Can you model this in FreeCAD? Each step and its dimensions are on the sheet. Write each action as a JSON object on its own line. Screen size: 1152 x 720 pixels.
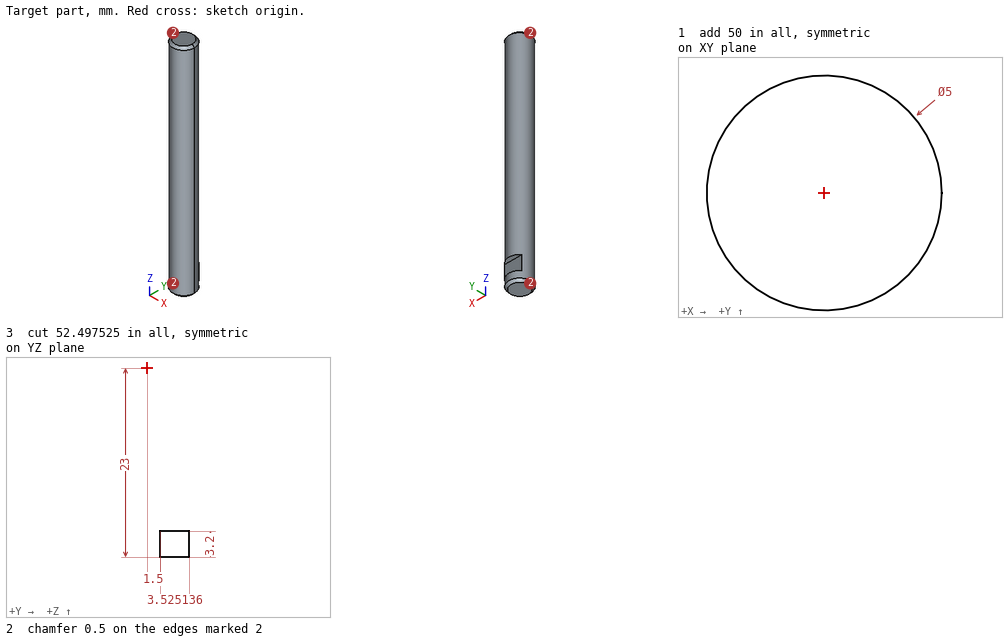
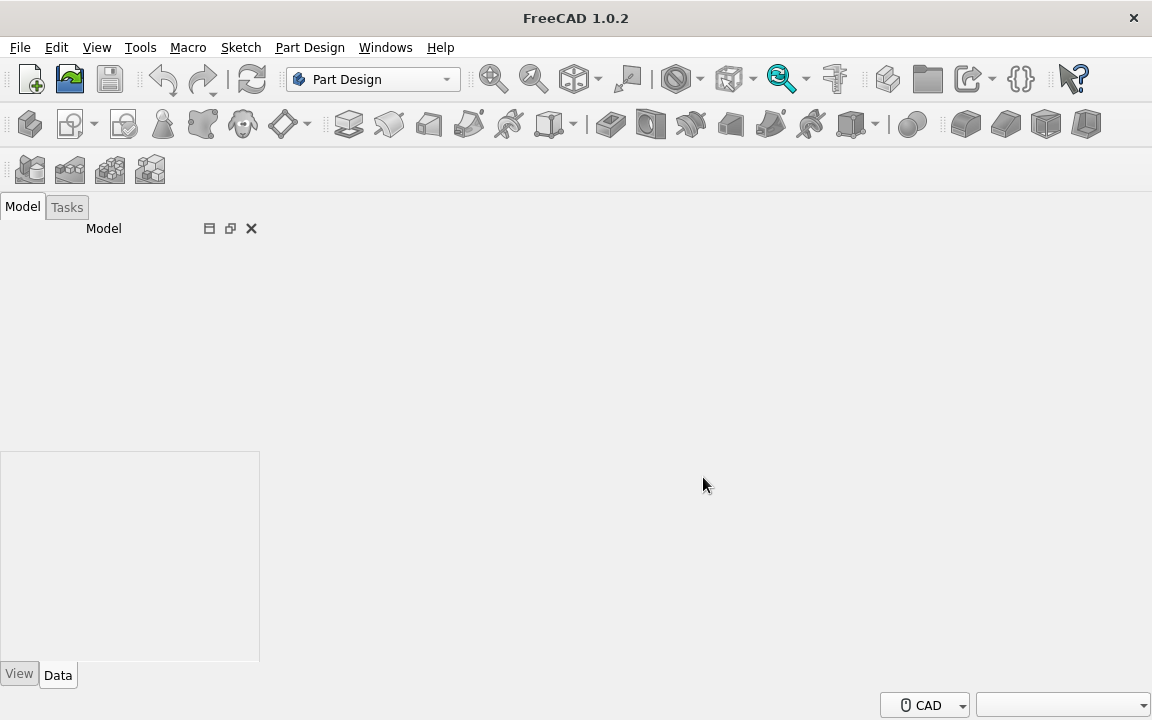
{"action": "left_click", "coordinate": [30, 80]}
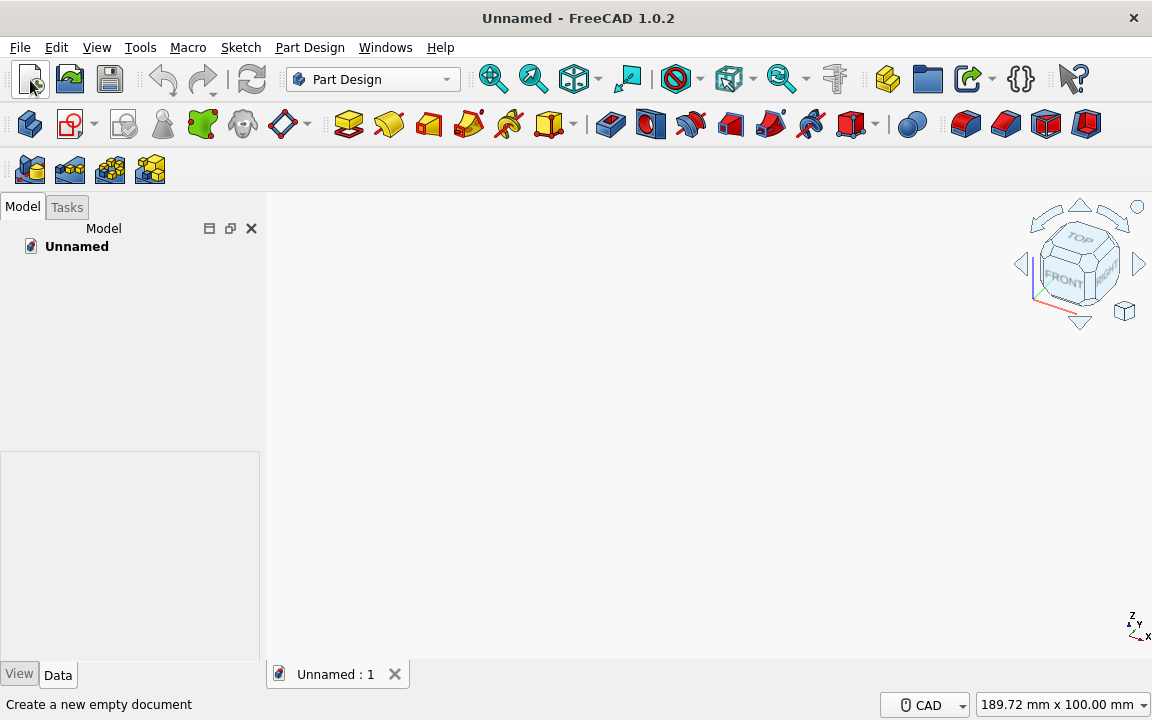
{"action": "left_click", "coordinate": [70, 124]}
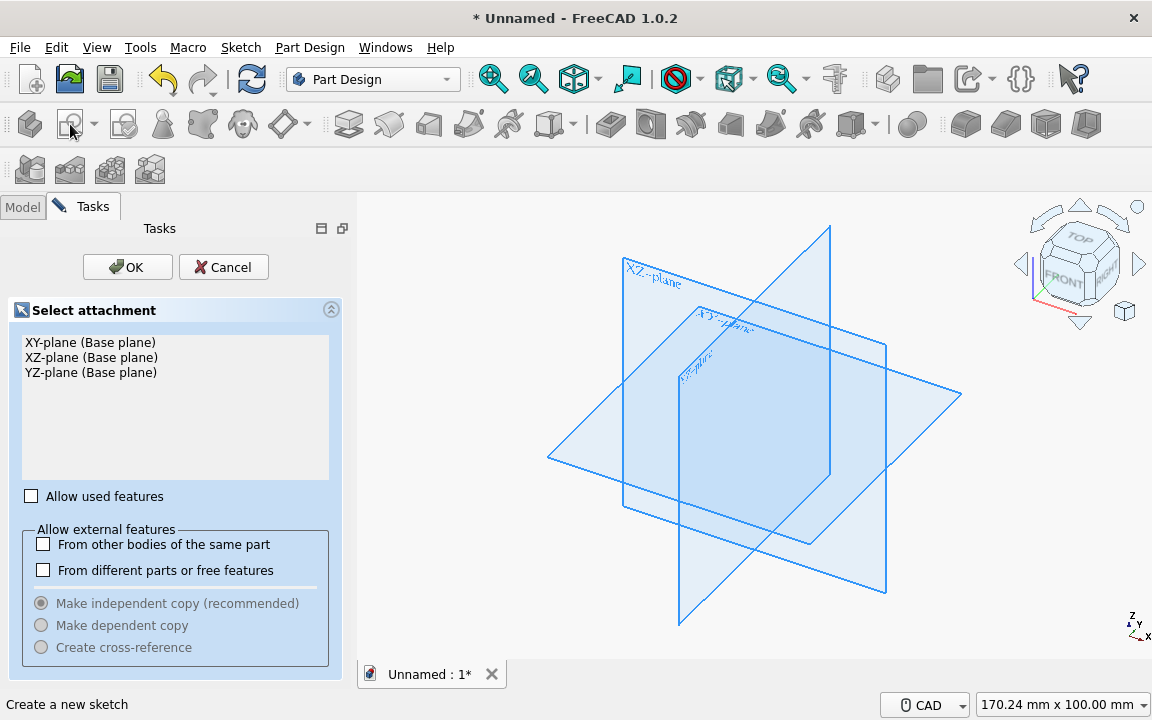
{"action": "left_click", "coordinate": [82, 342]}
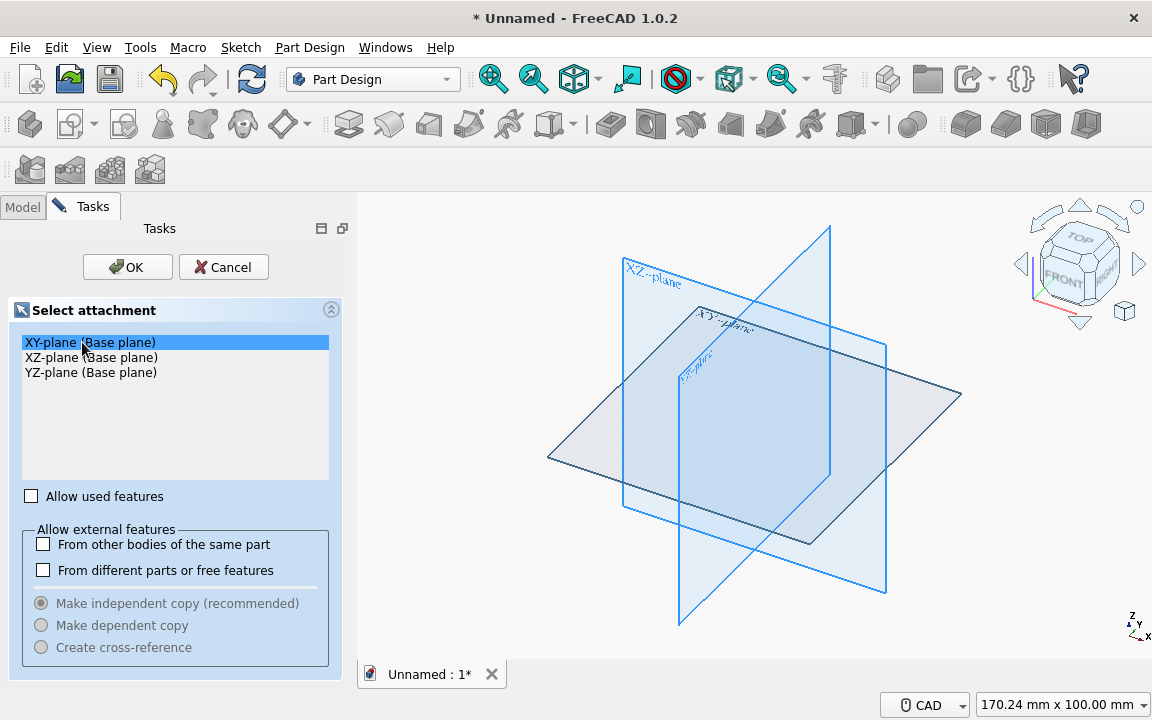
{"action": "left_click", "coordinate": [128, 267]}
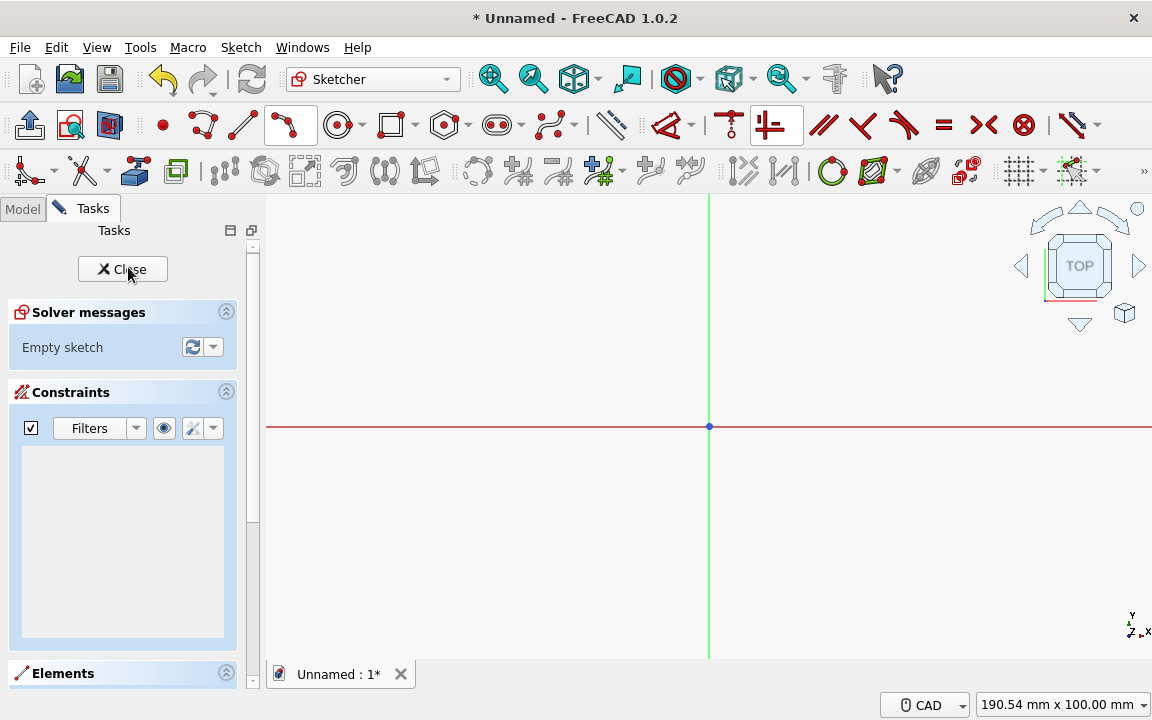
{"action": "scroll", "coordinate": [714, 426], "scroll_direction": "up", "scroll_amount": 13}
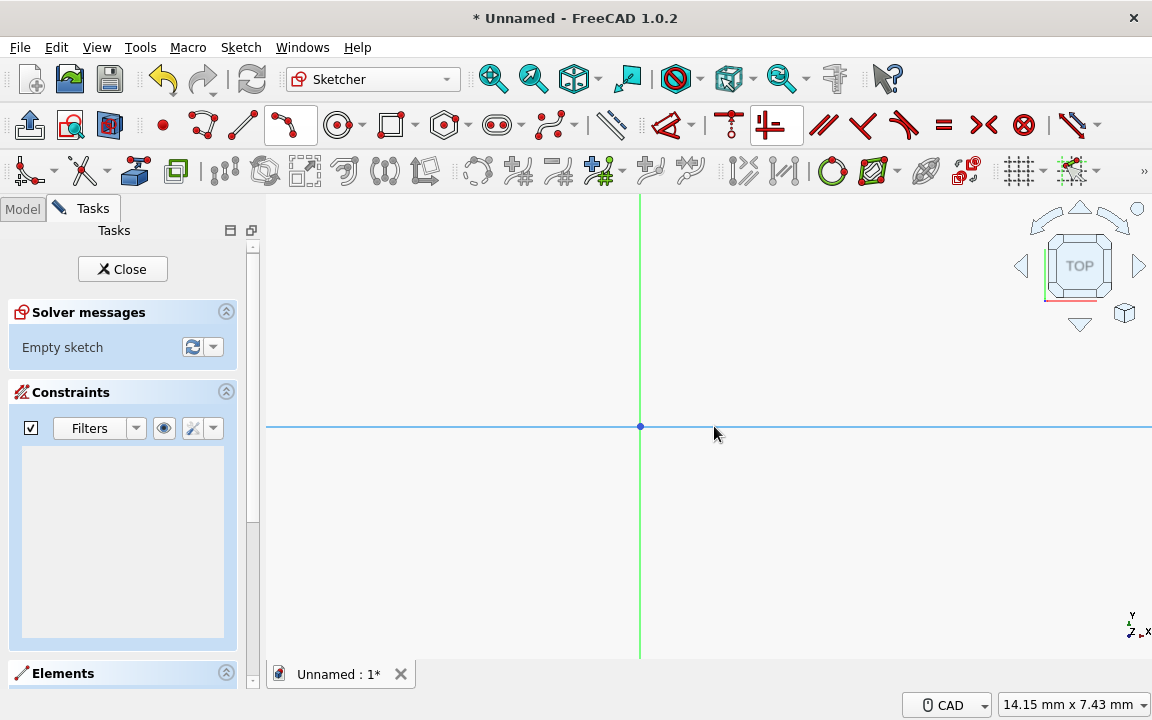
{"action": "key", "text": "g c"}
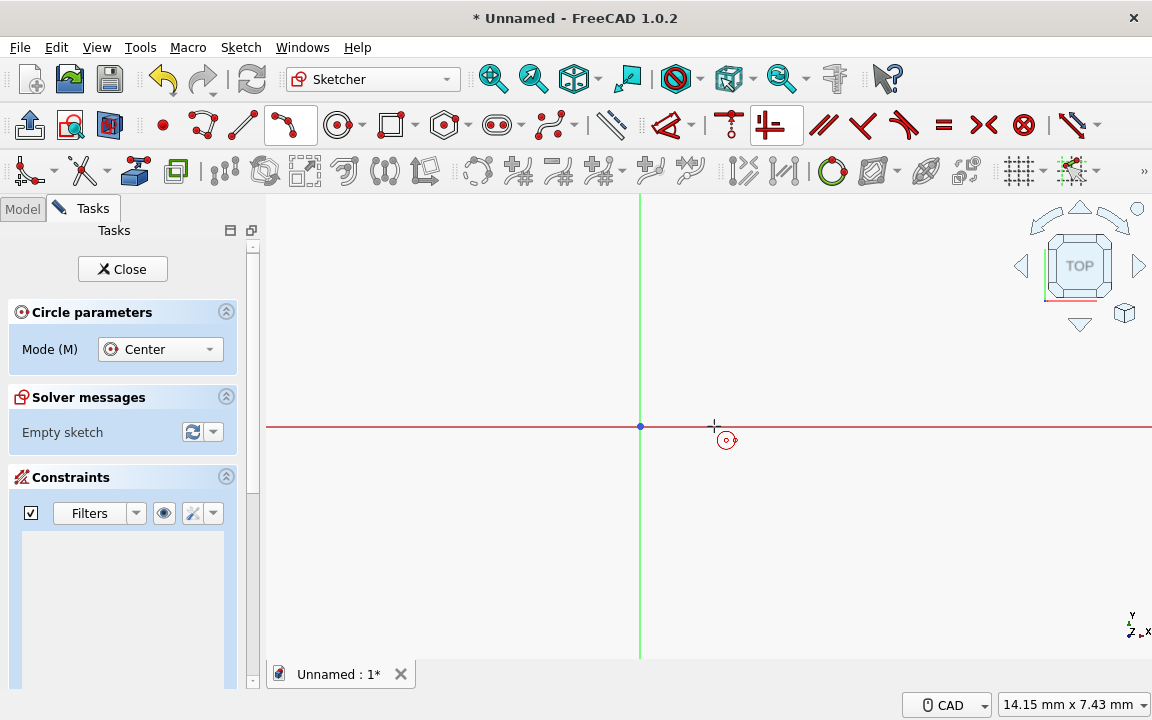
{"action": "left_click", "coordinate": [640, 426]}
{"action": "mouse_move", "coordinate": [751, 316]}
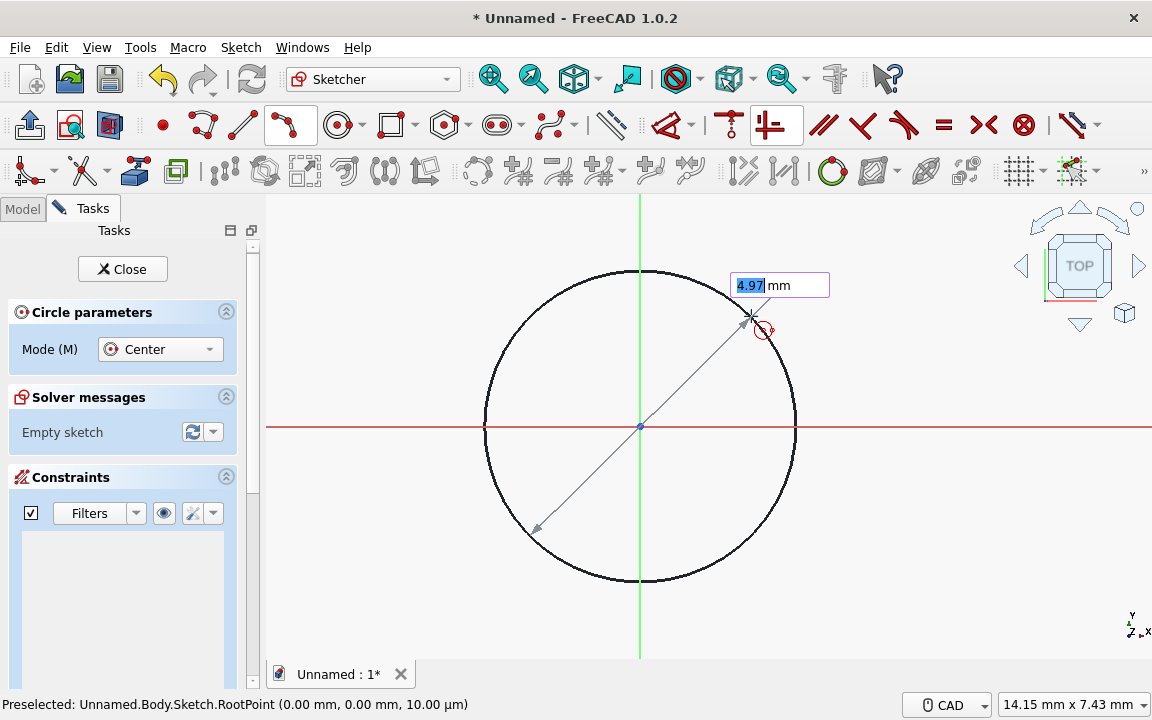
{"action": "type", "text": "5"}
{"action": "key", "text": "Return"}
{"action": "key", "text": "Escape"}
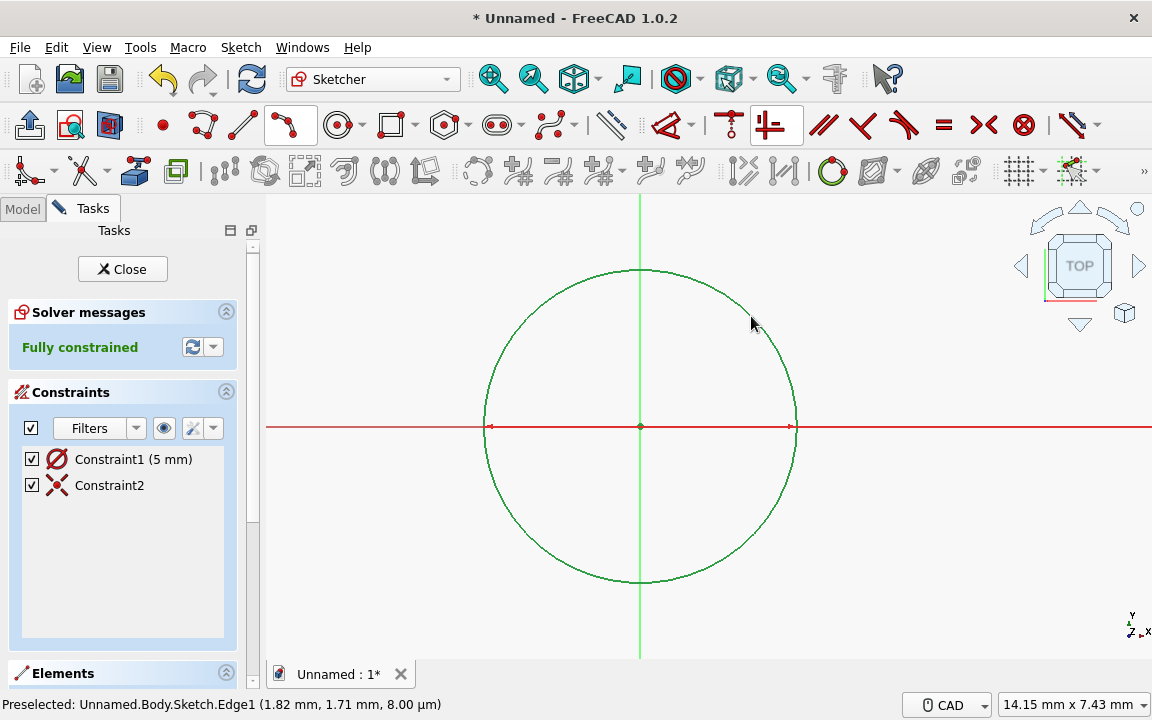
{"action": "left_click", "coordinate": [123, 269]}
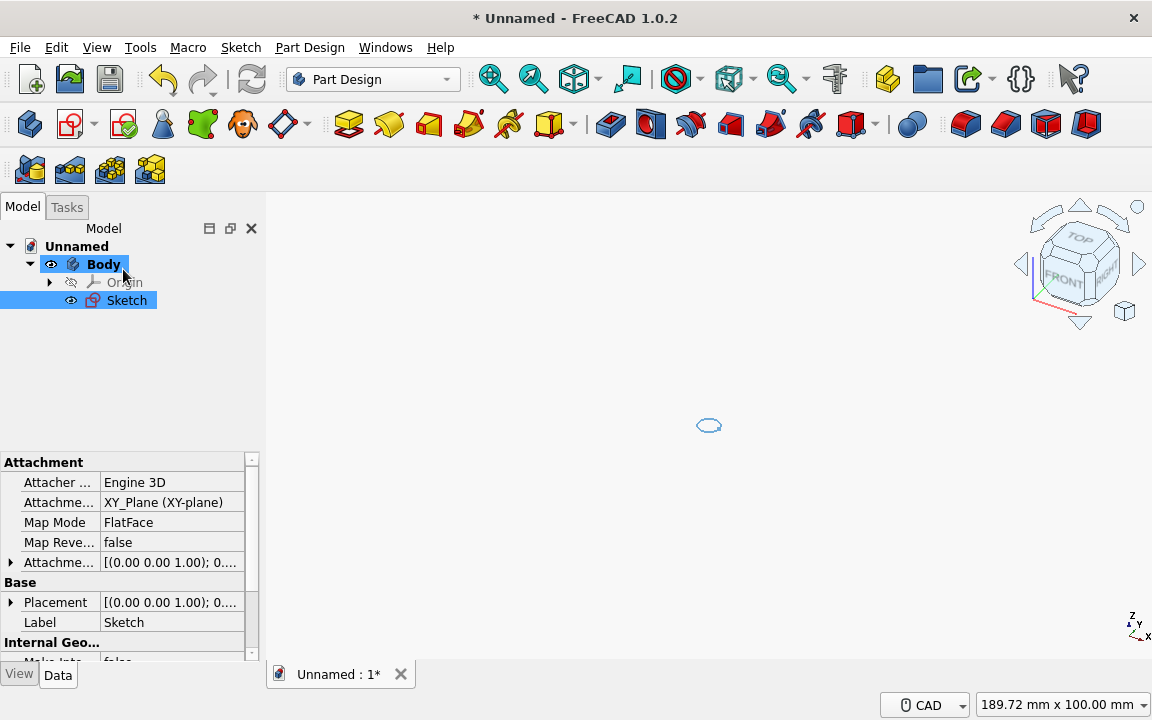
{"action": "left_click", "coordinate": [350, 124]}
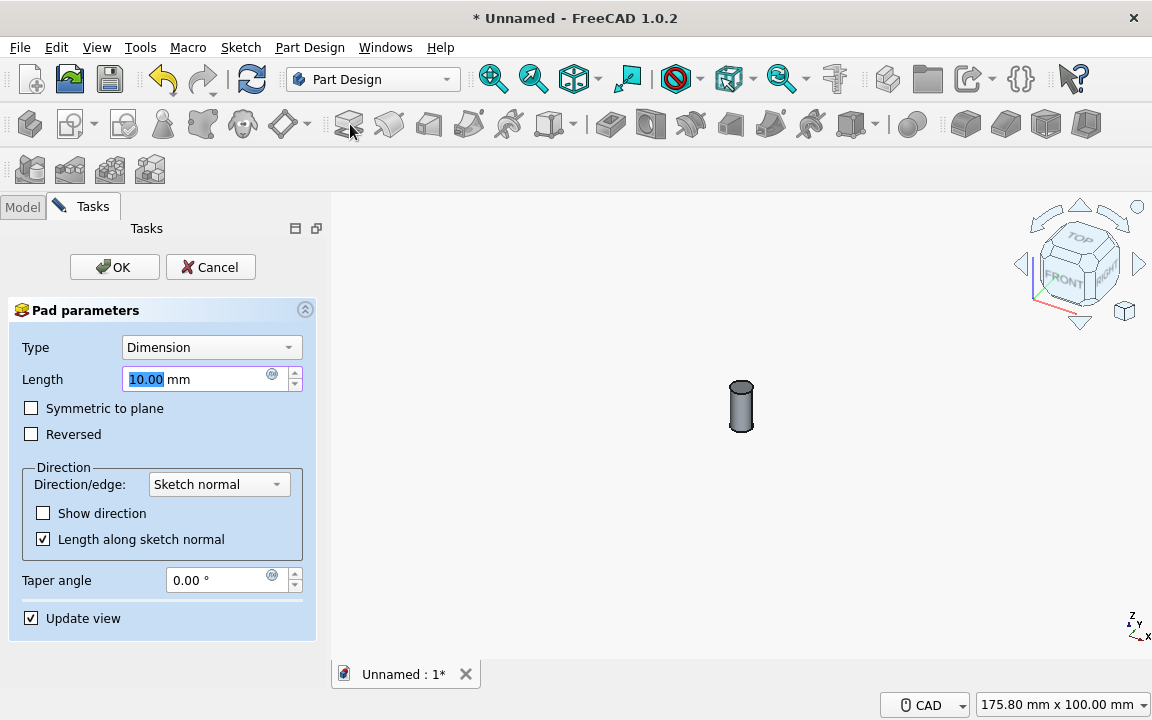
{"action": "type", "text": "50"}
{"action": "key", "text": "Tab"}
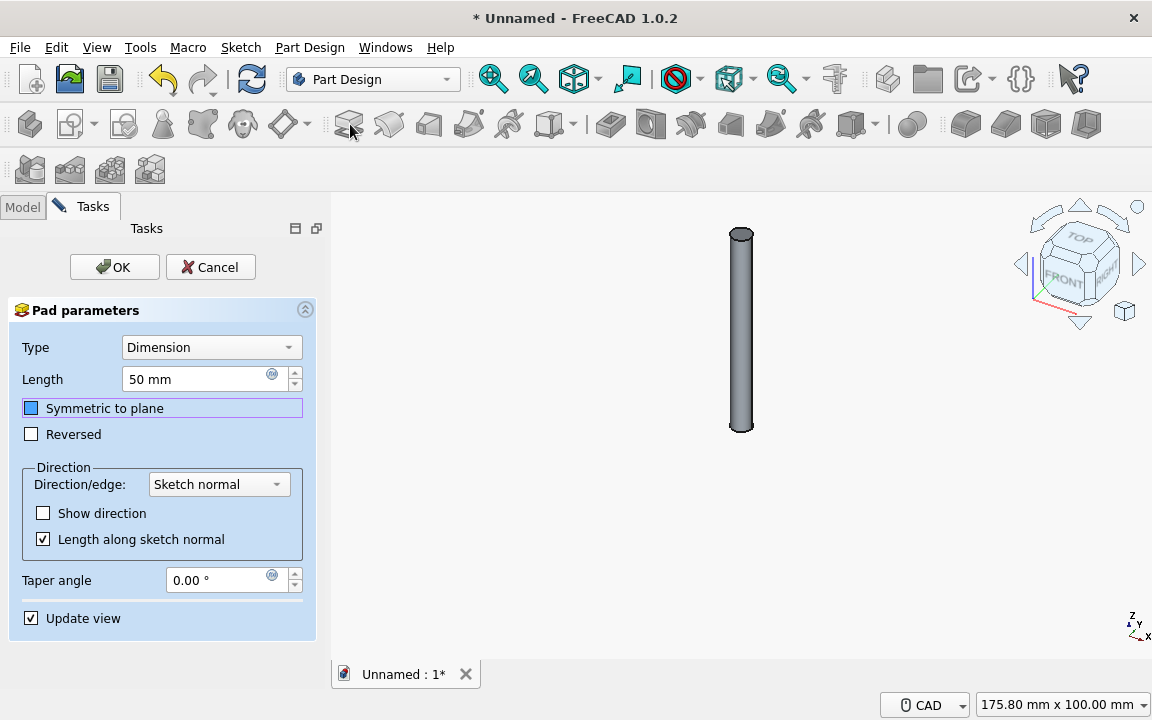
{"action": "left_click", "coordinate": [30, 408]}